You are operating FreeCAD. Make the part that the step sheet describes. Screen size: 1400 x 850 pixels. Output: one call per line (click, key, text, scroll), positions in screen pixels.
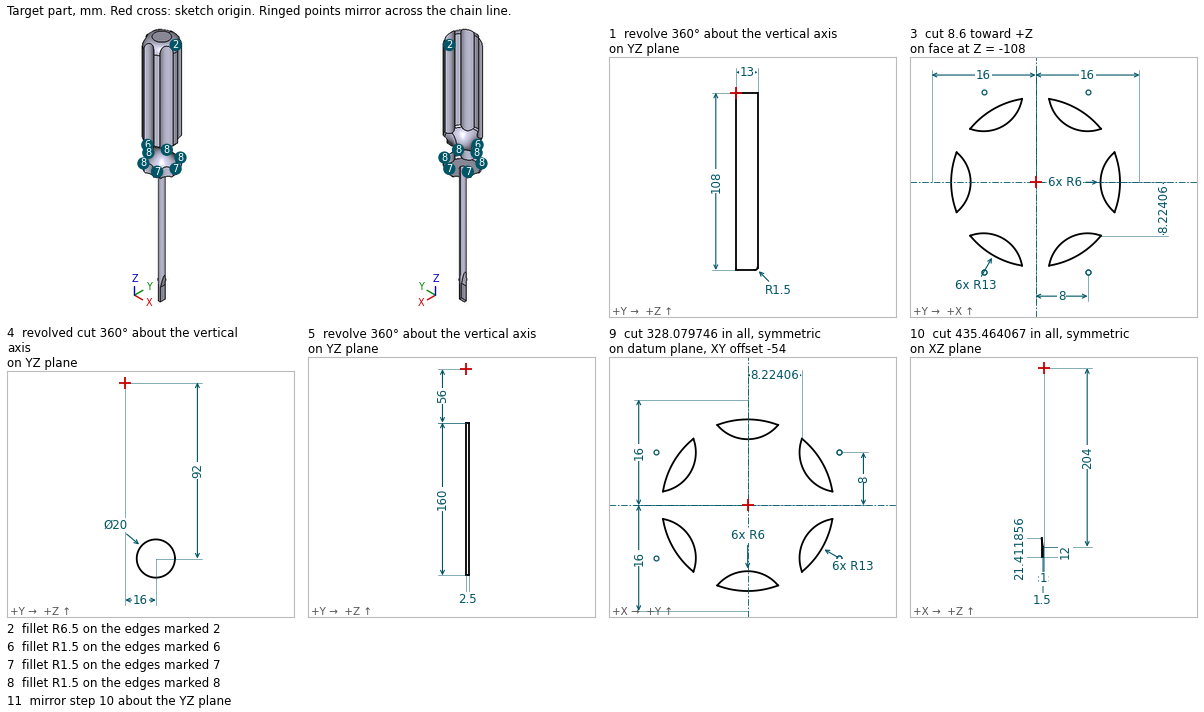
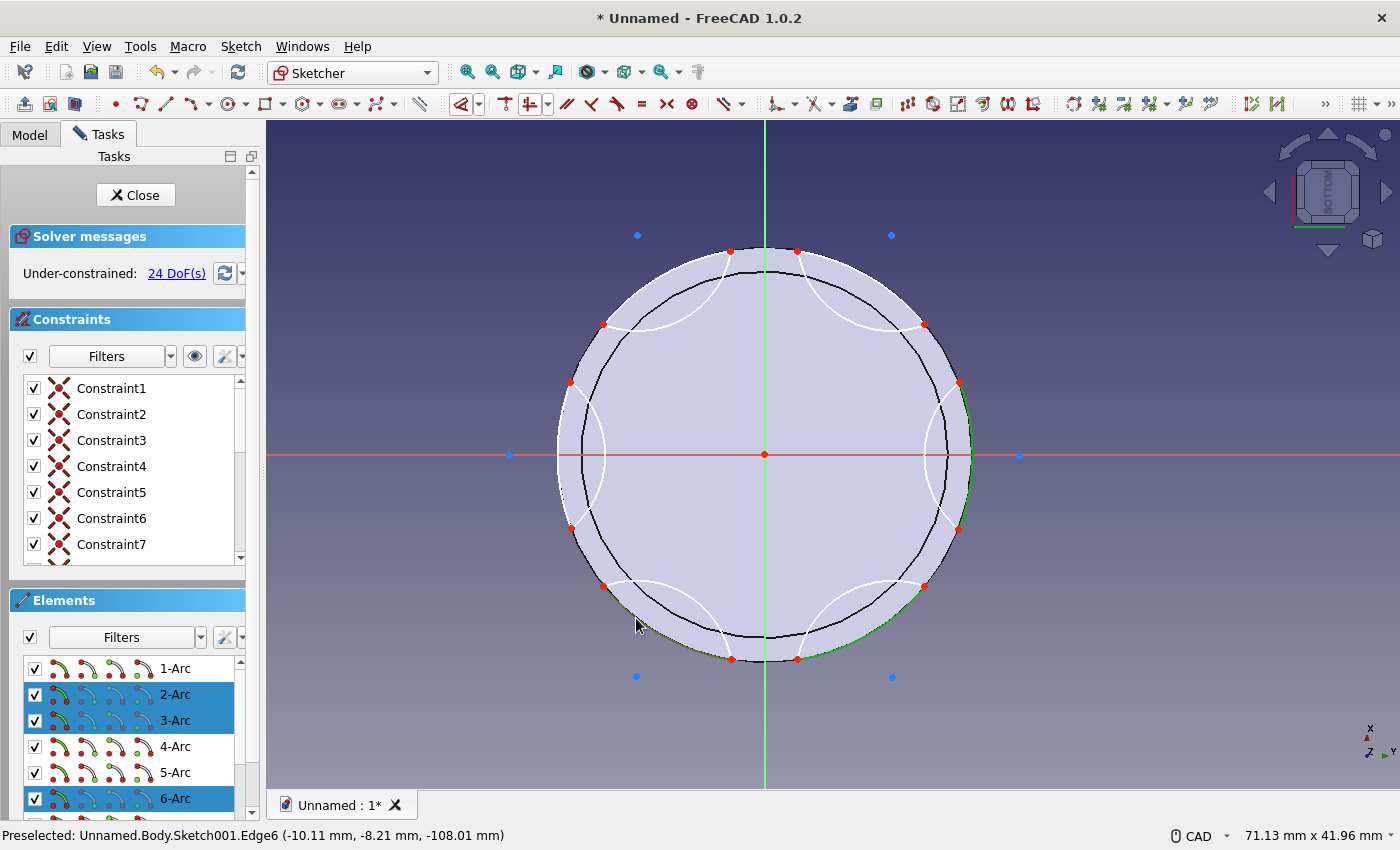
click(560, 426)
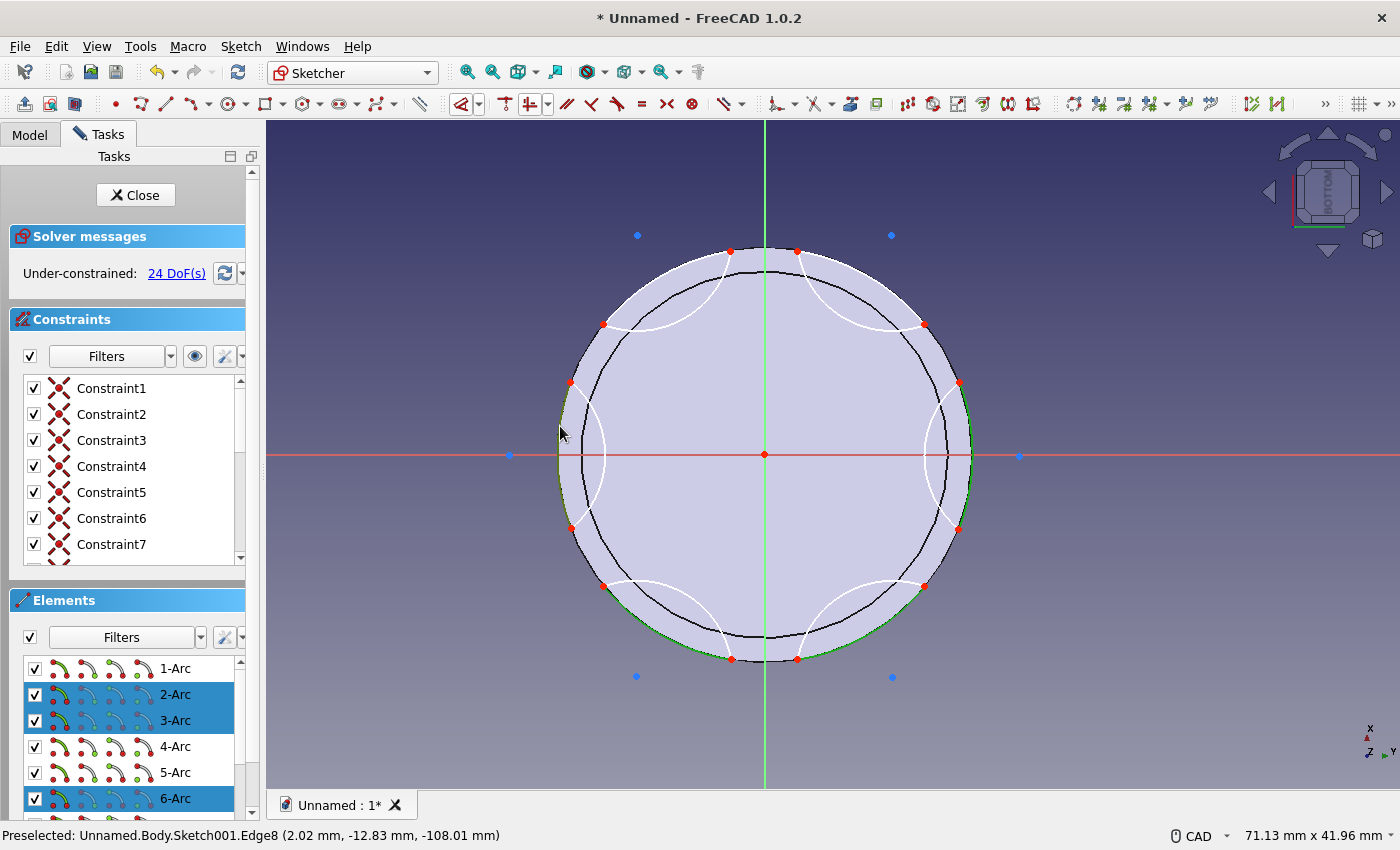
click(688, 263)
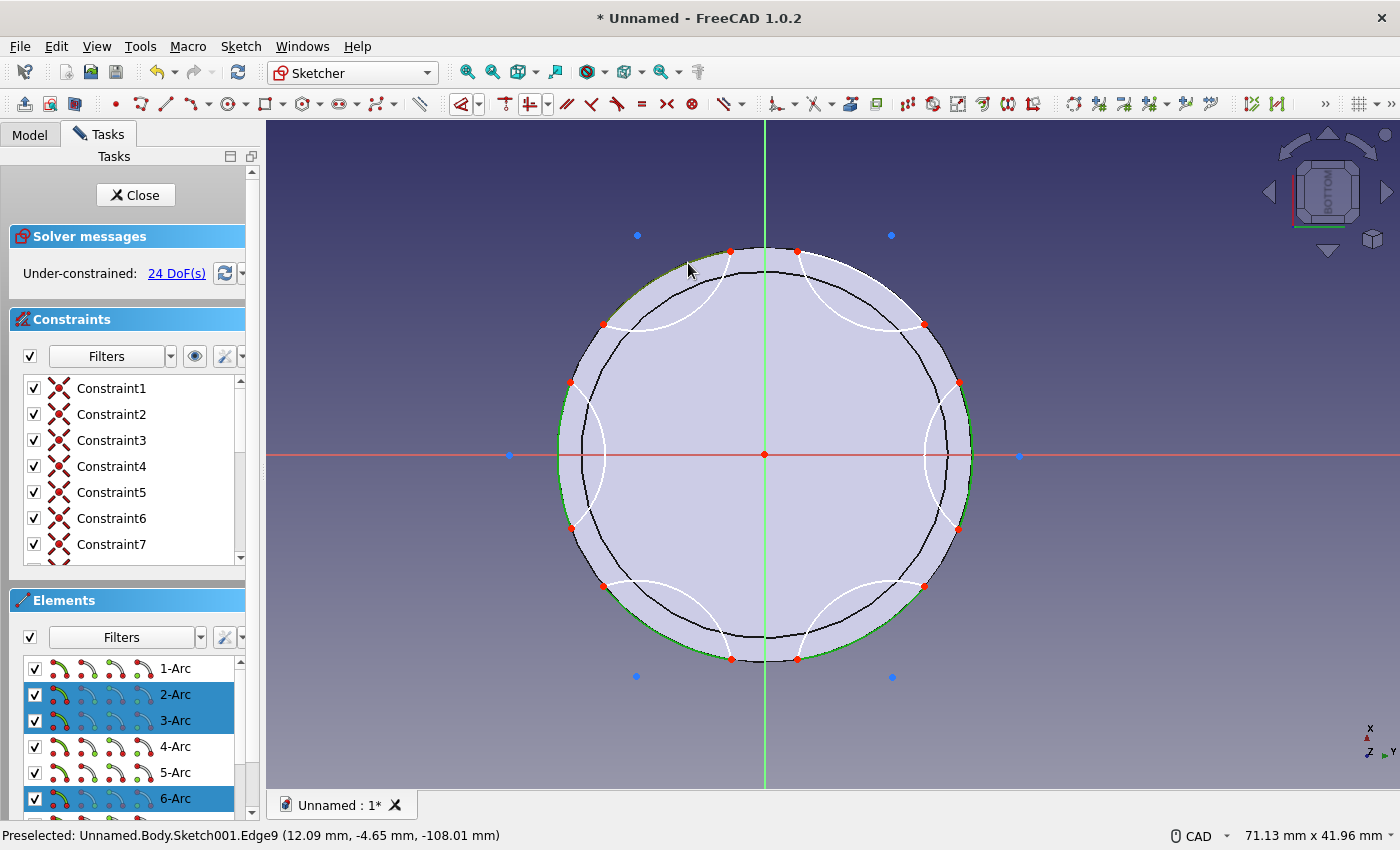
click(893, 293)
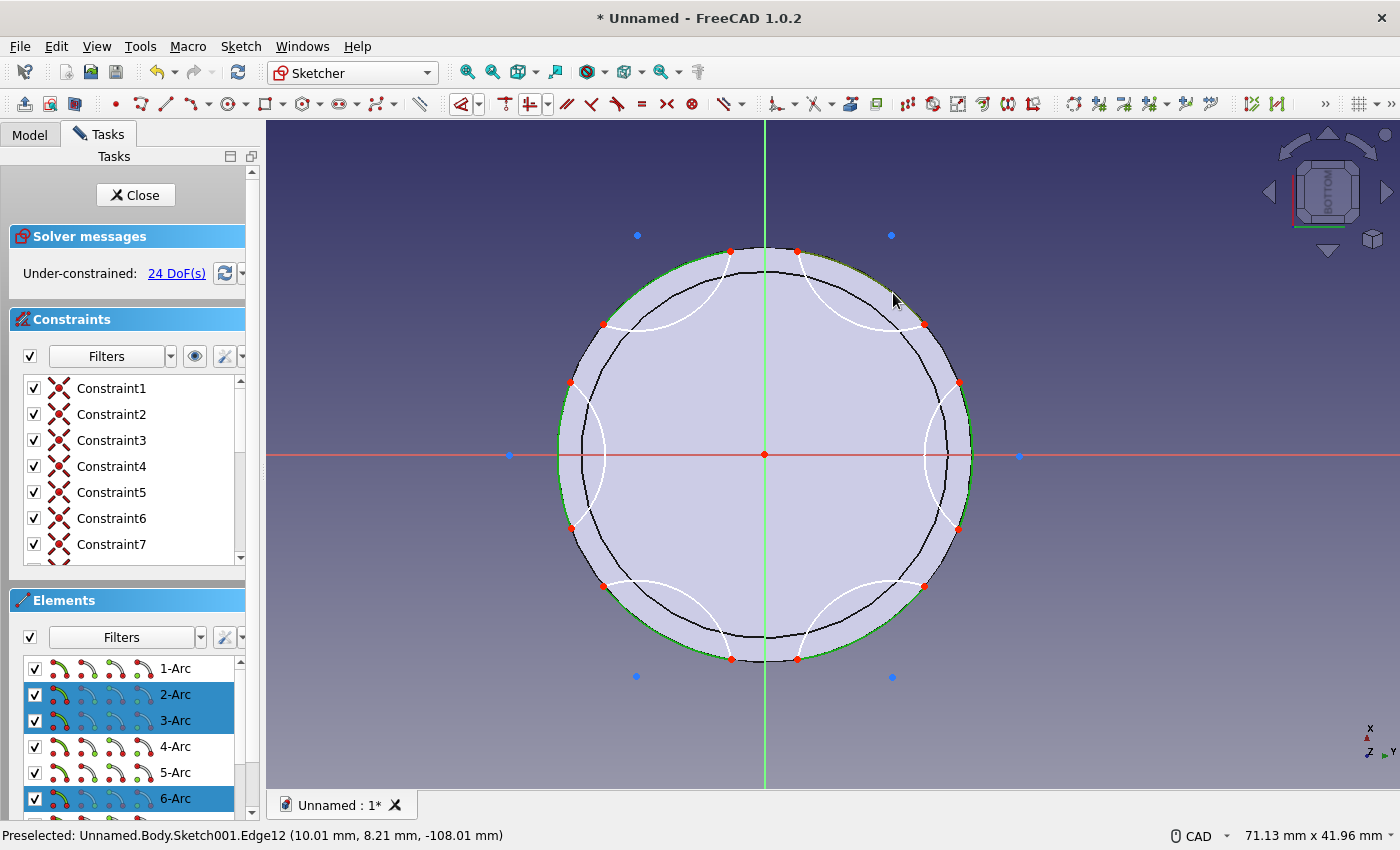
click(642, 104)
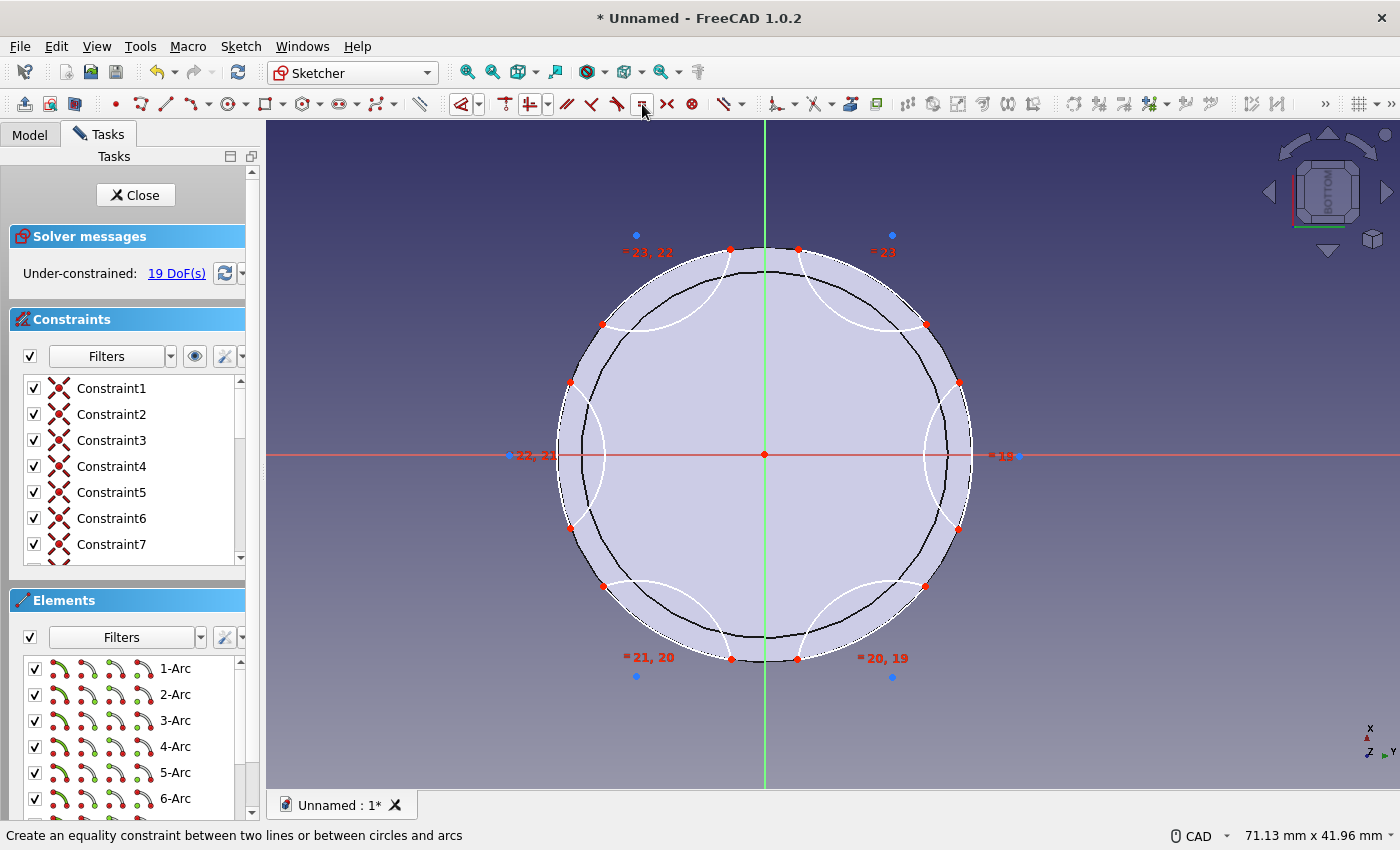
click(930, 423)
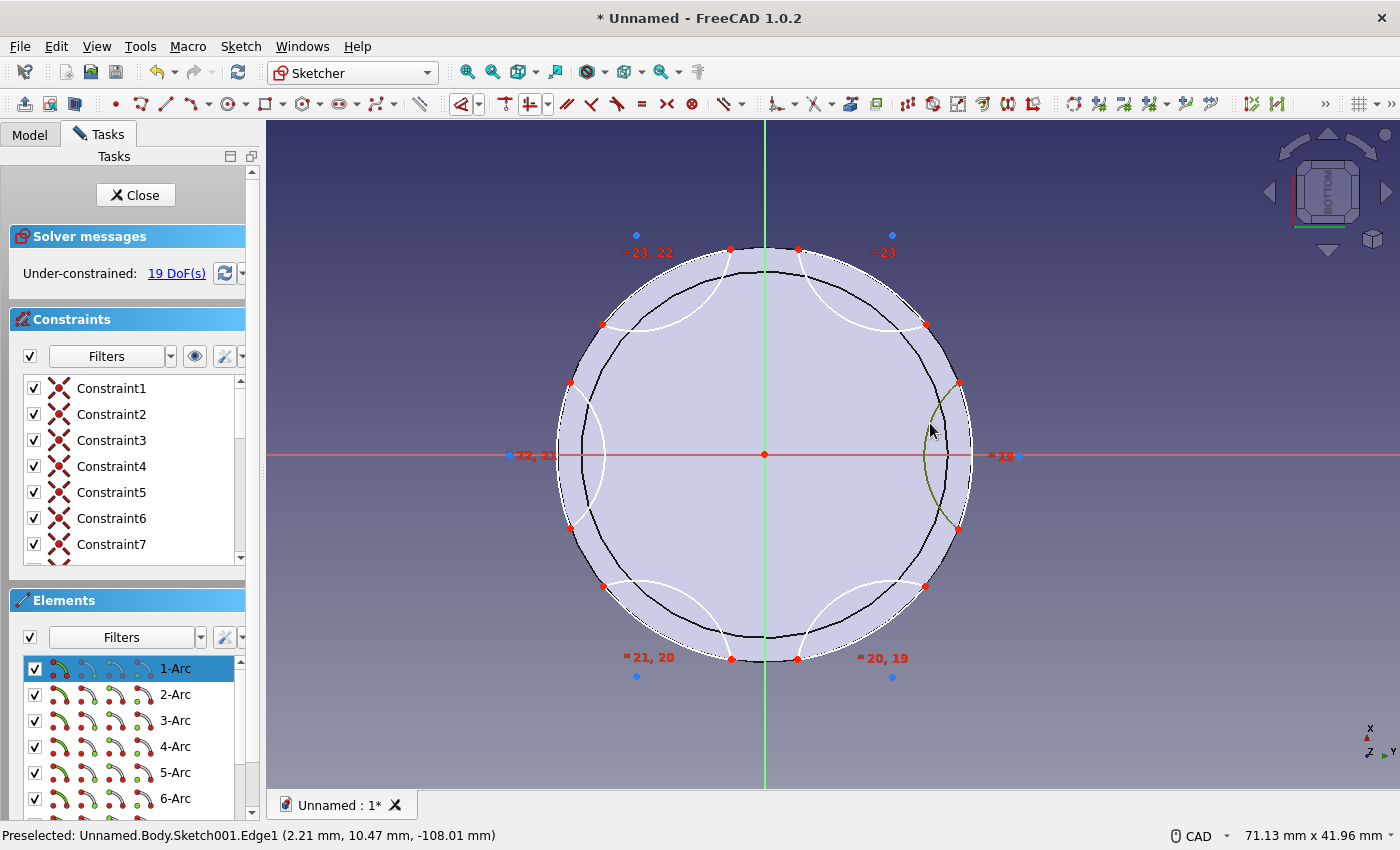
click(876, 582)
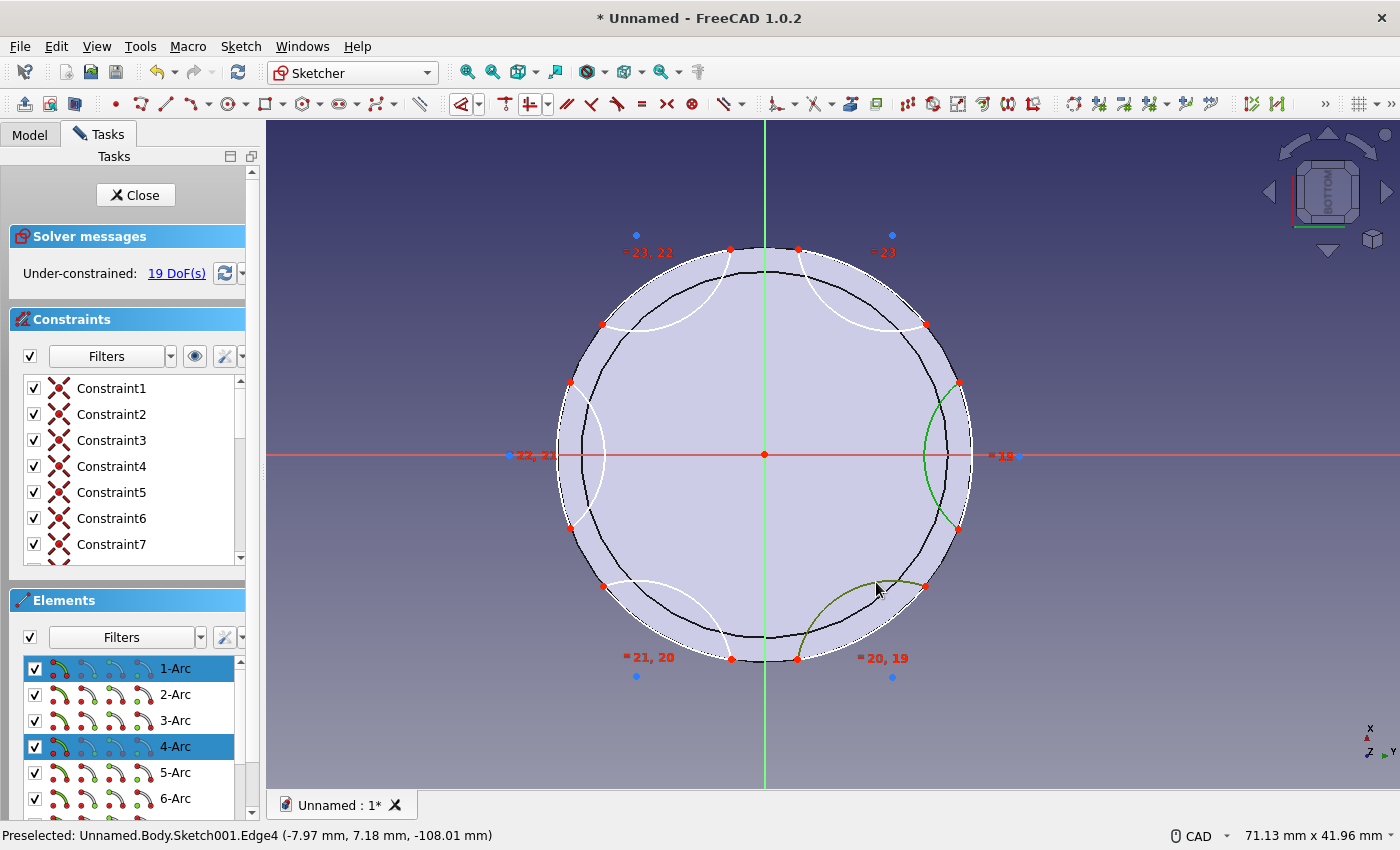
click(710, 615)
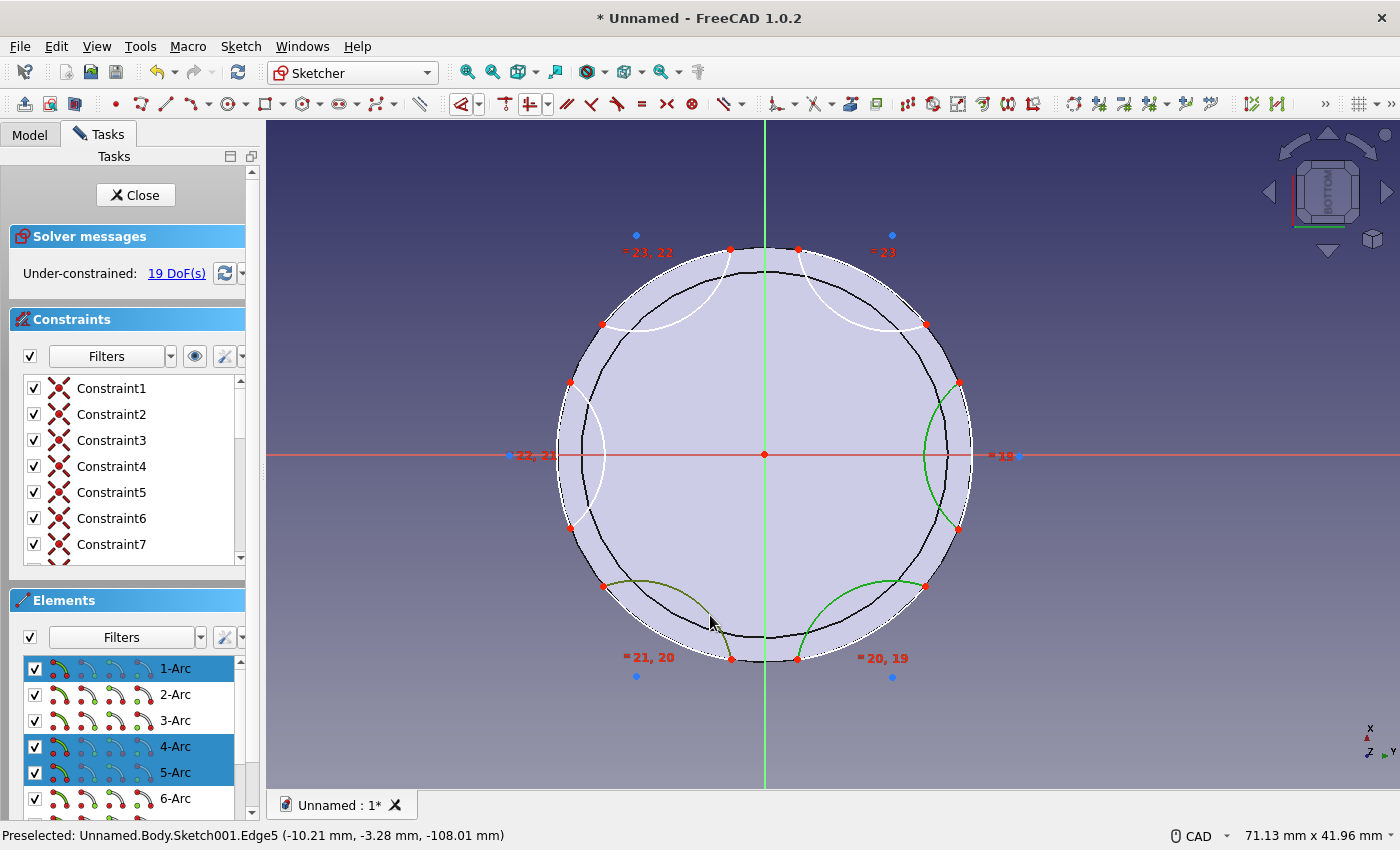
click(599, 488)